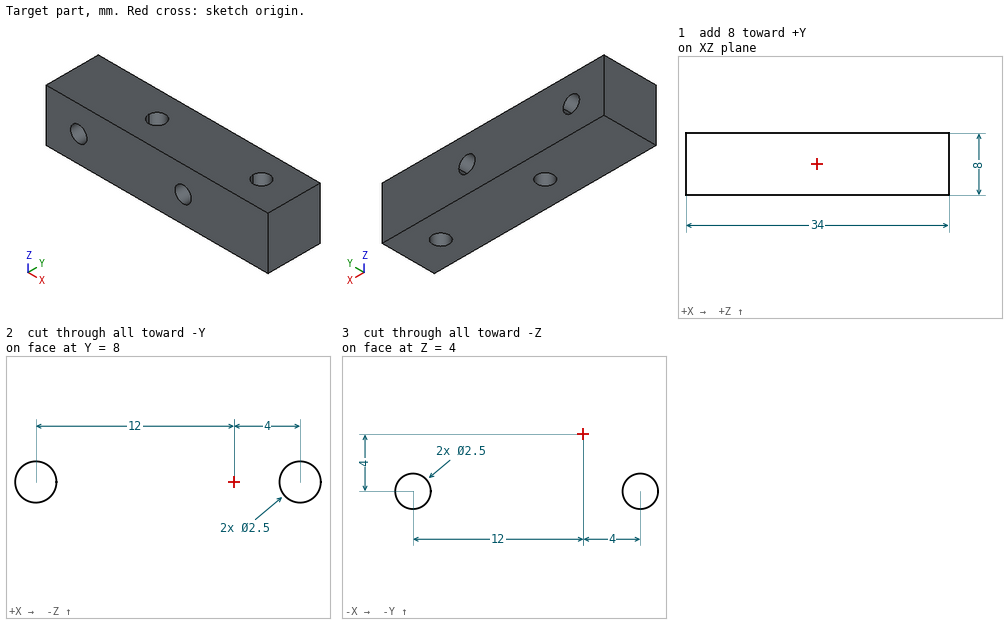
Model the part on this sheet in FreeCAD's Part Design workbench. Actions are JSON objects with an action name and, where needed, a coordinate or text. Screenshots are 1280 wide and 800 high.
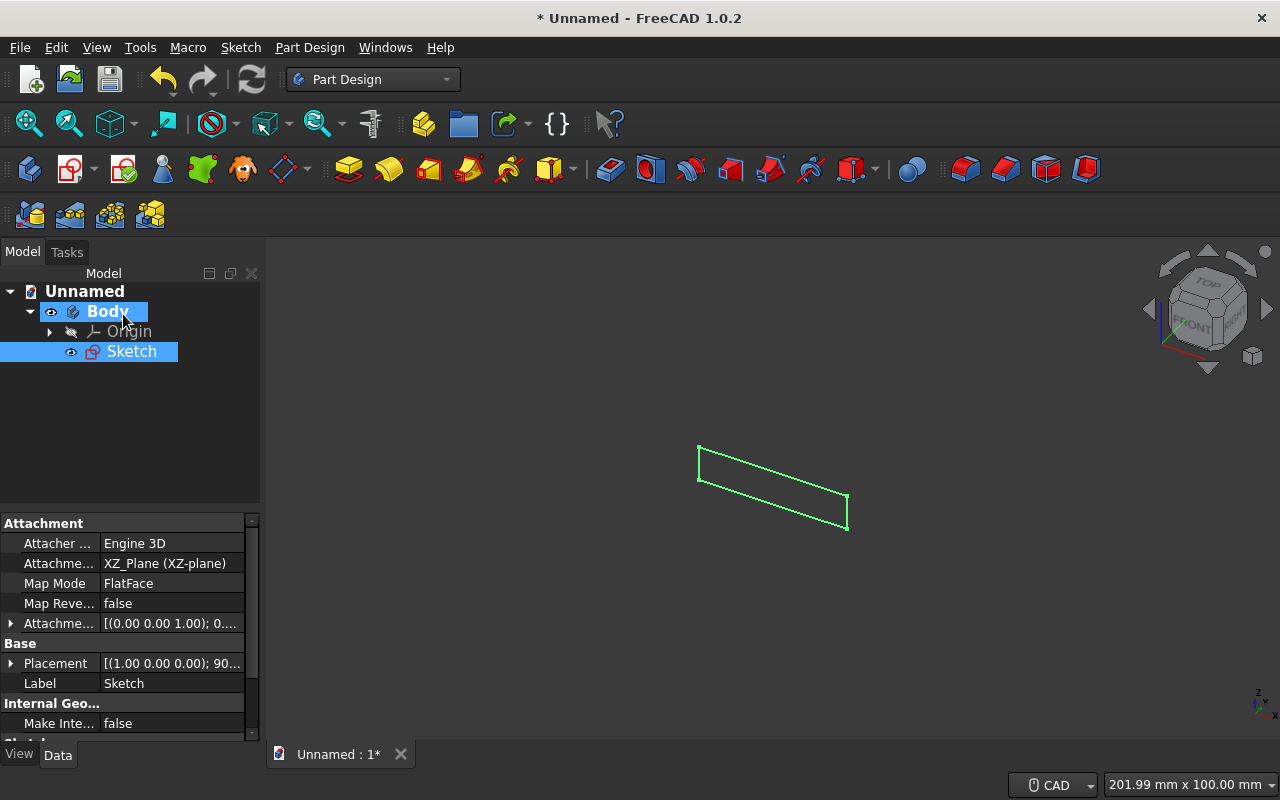
{"action": "left_click", "coordinate": [350, 170]}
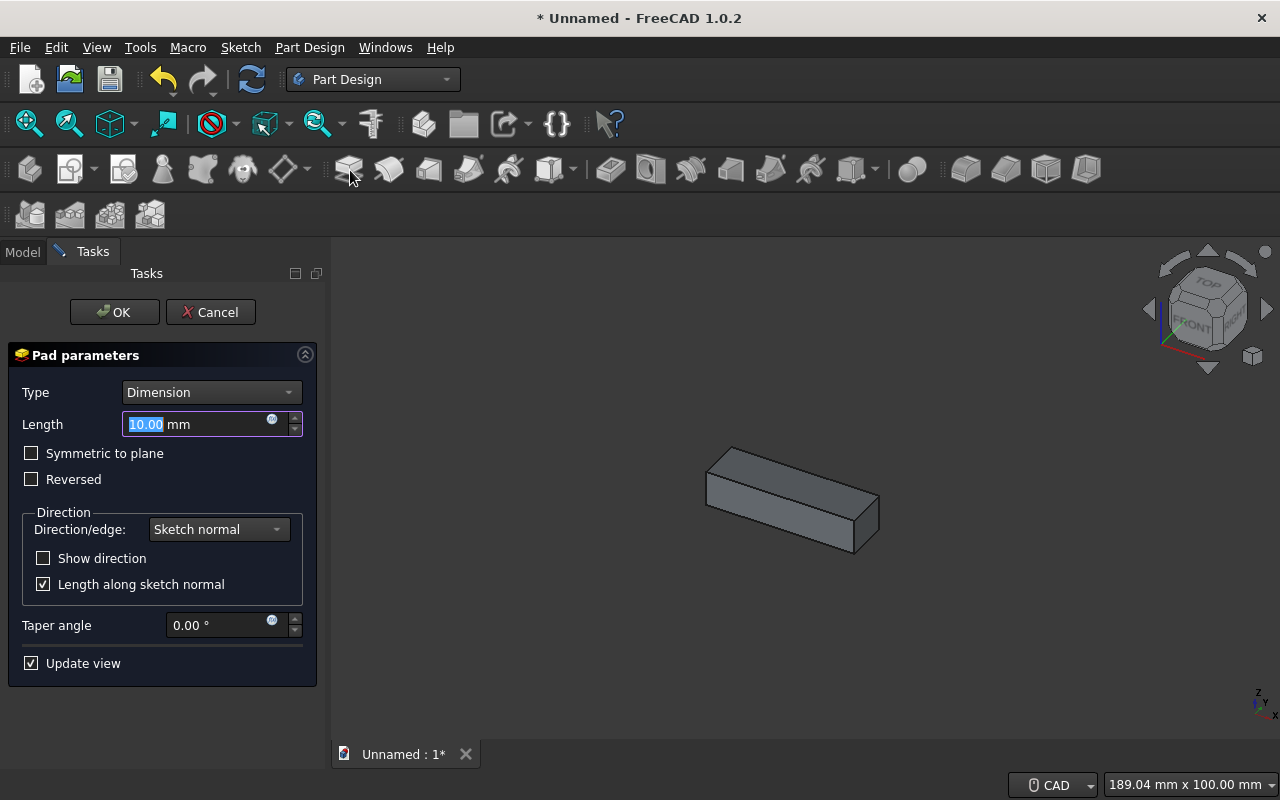
{"action": "type", "text": "8"}
{"action": "key", "text": "Tab"}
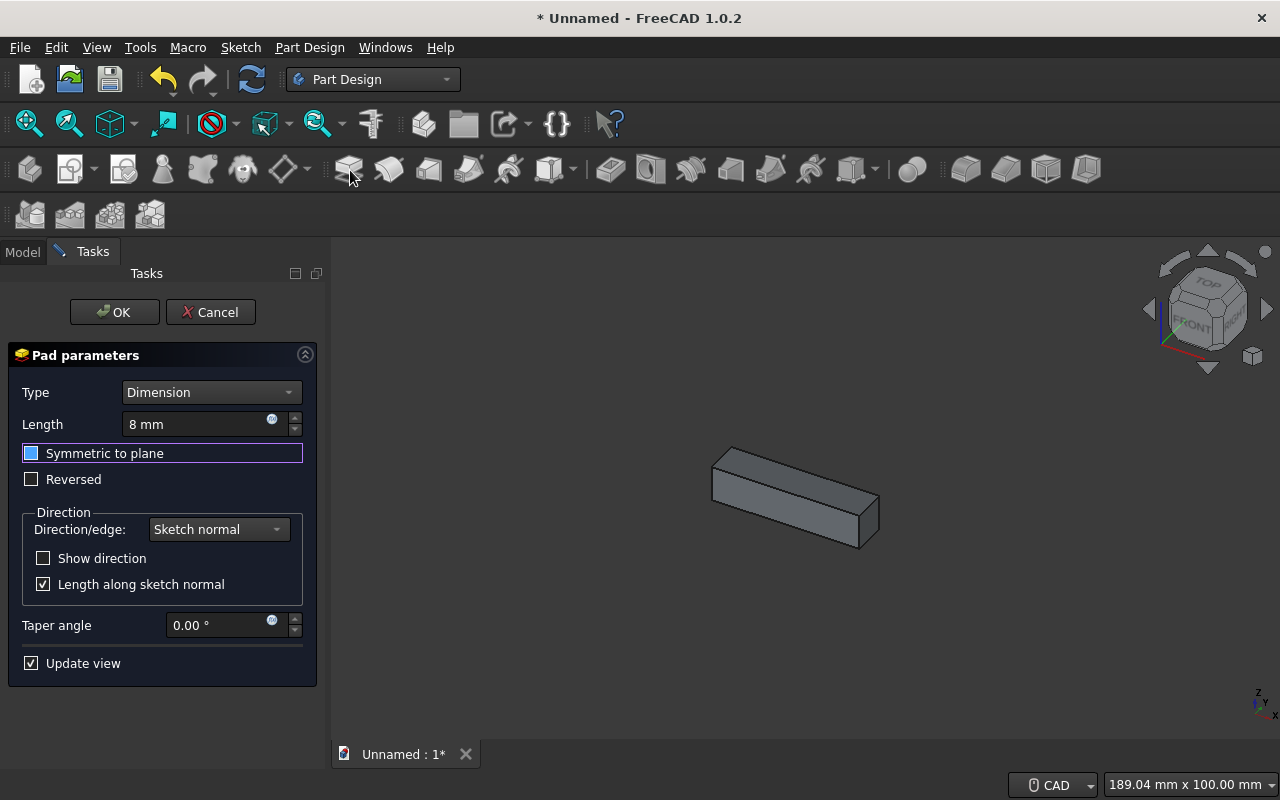
{"action": "left_click", "coordinate": [30, 479]}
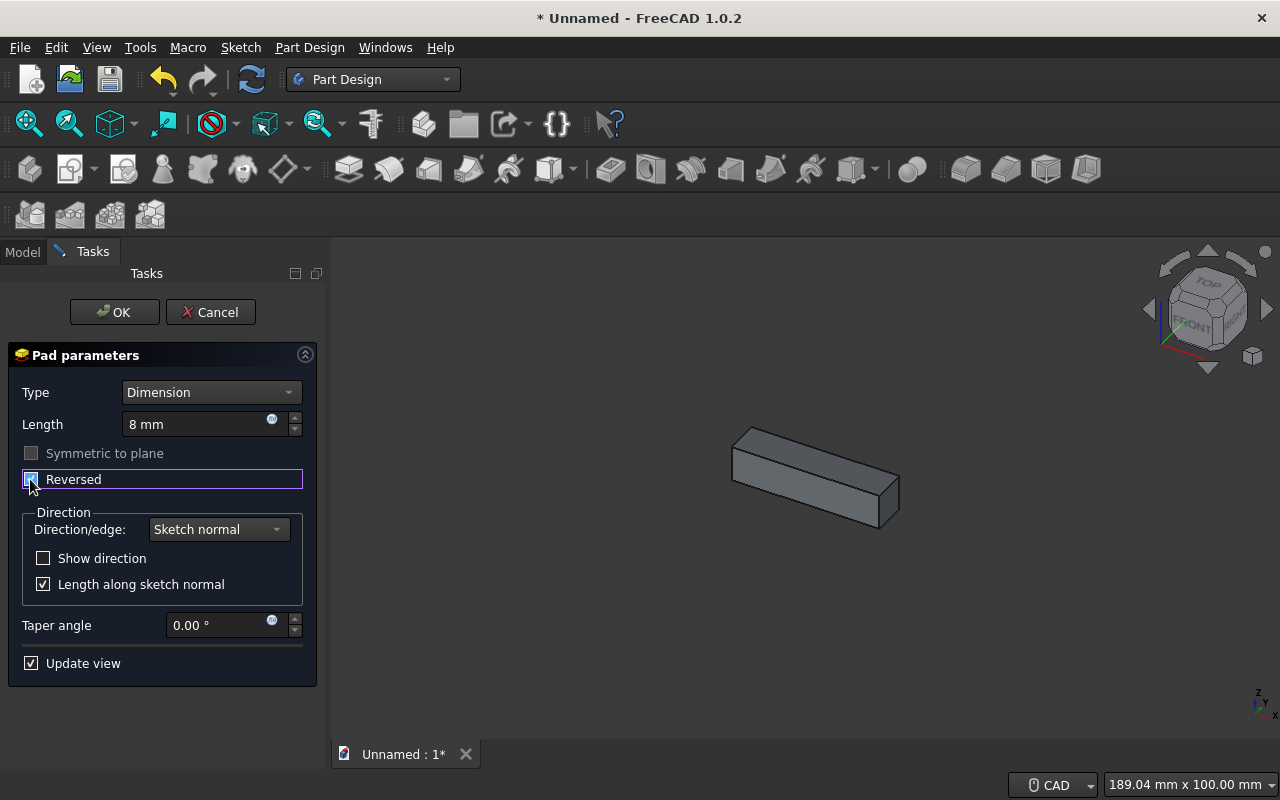
{"action": "left_click", "coordinate": [115, 312]}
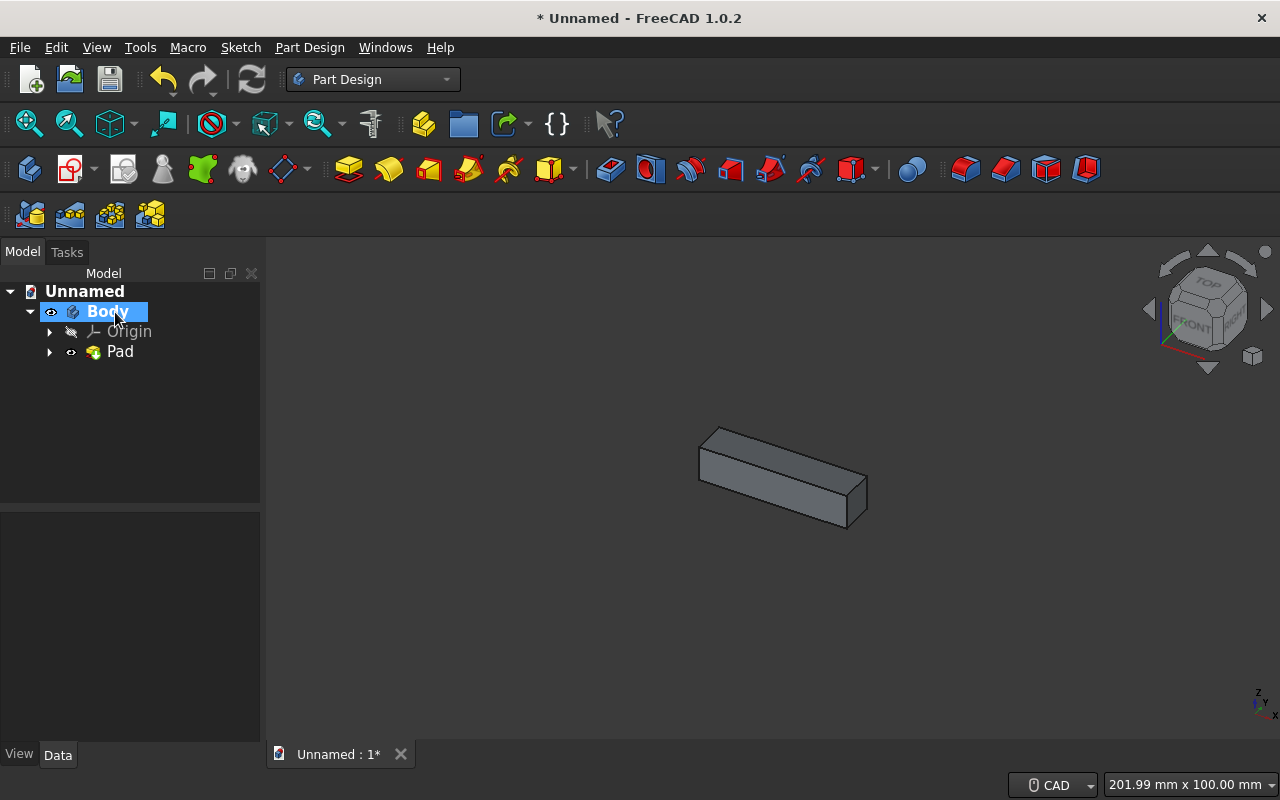
{"action": "left_click", "coordinate": [30, 124]}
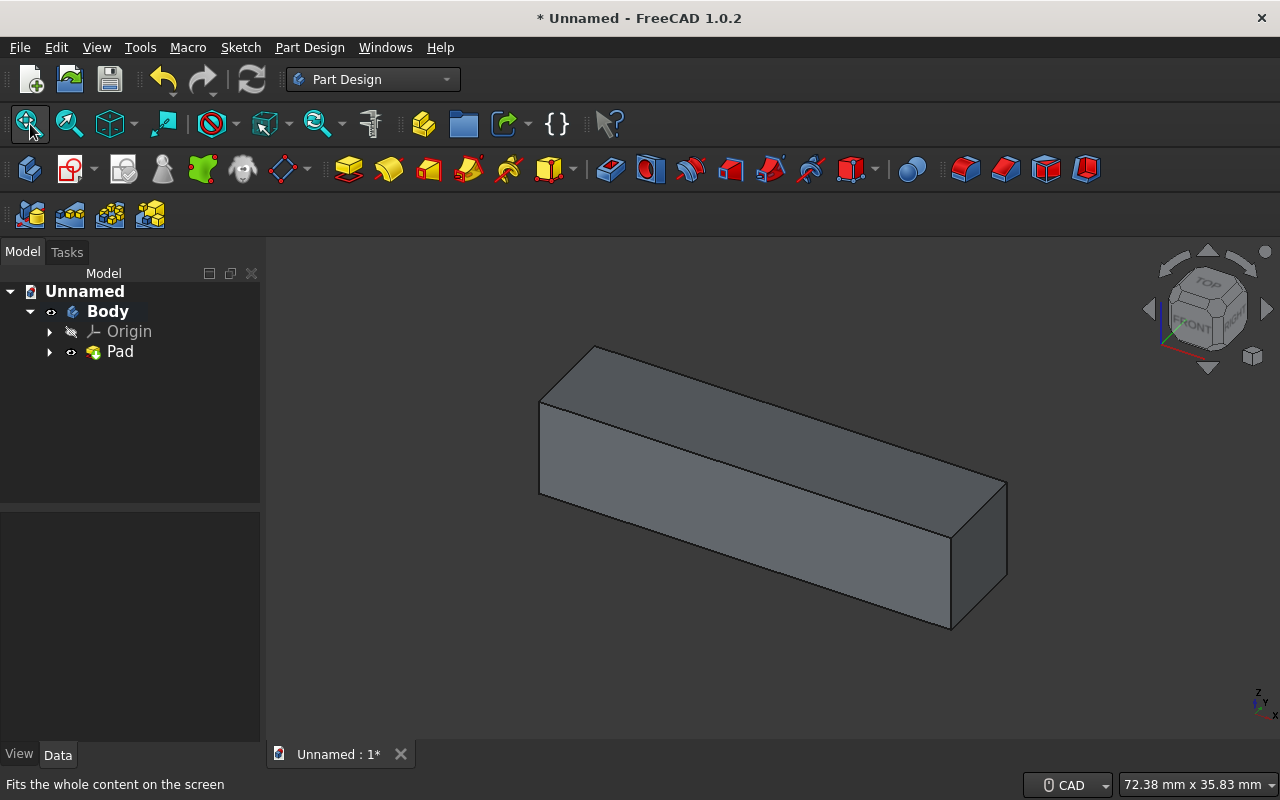
{"action": "key", "text": "4"}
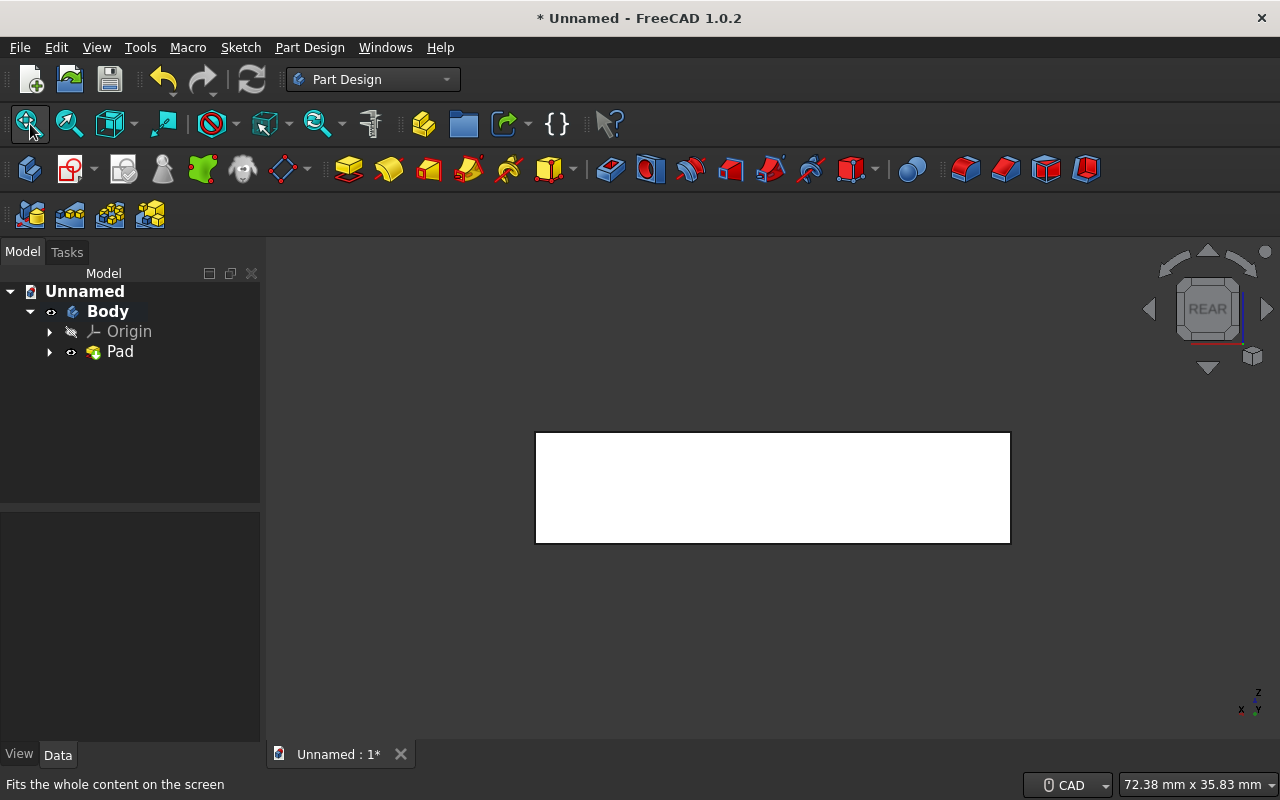
{"action": "left_click", "coordinate": [637, 487]}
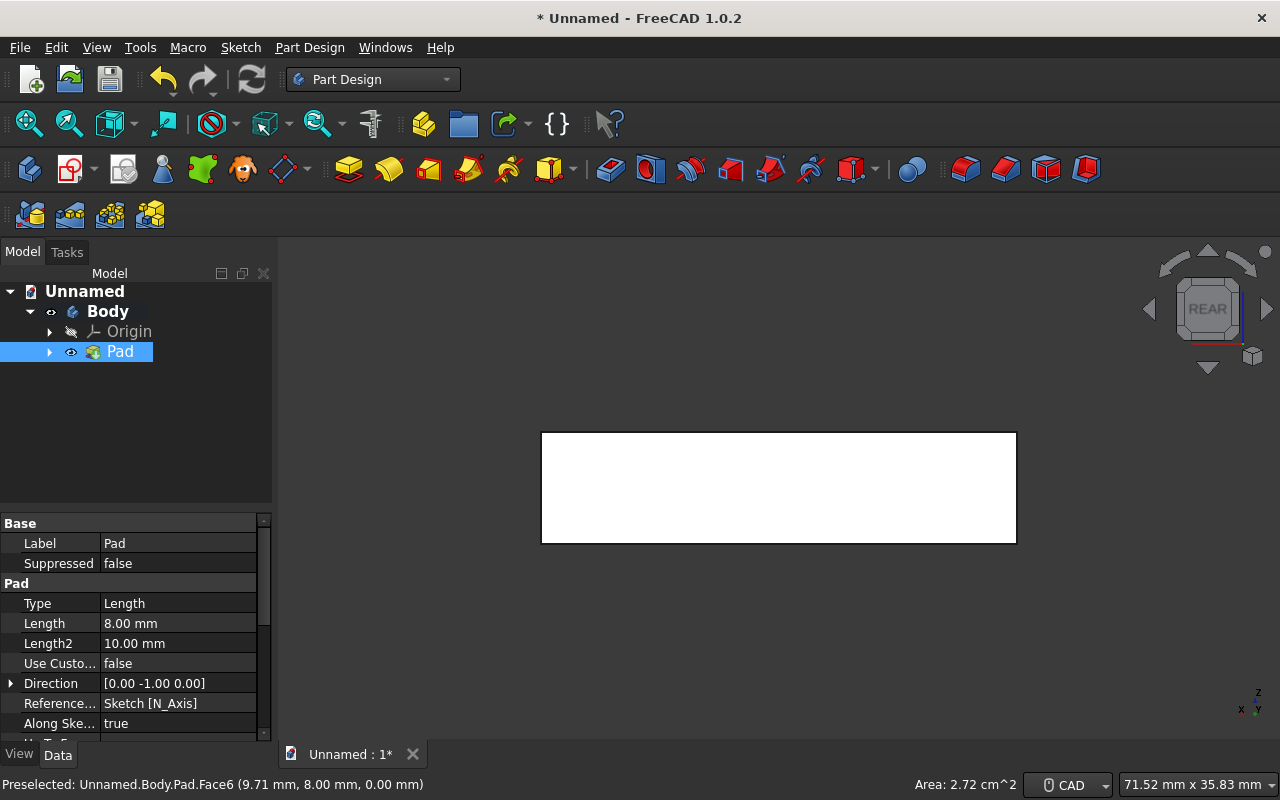
{"action": "left_click", "coordinate": [70, 170]}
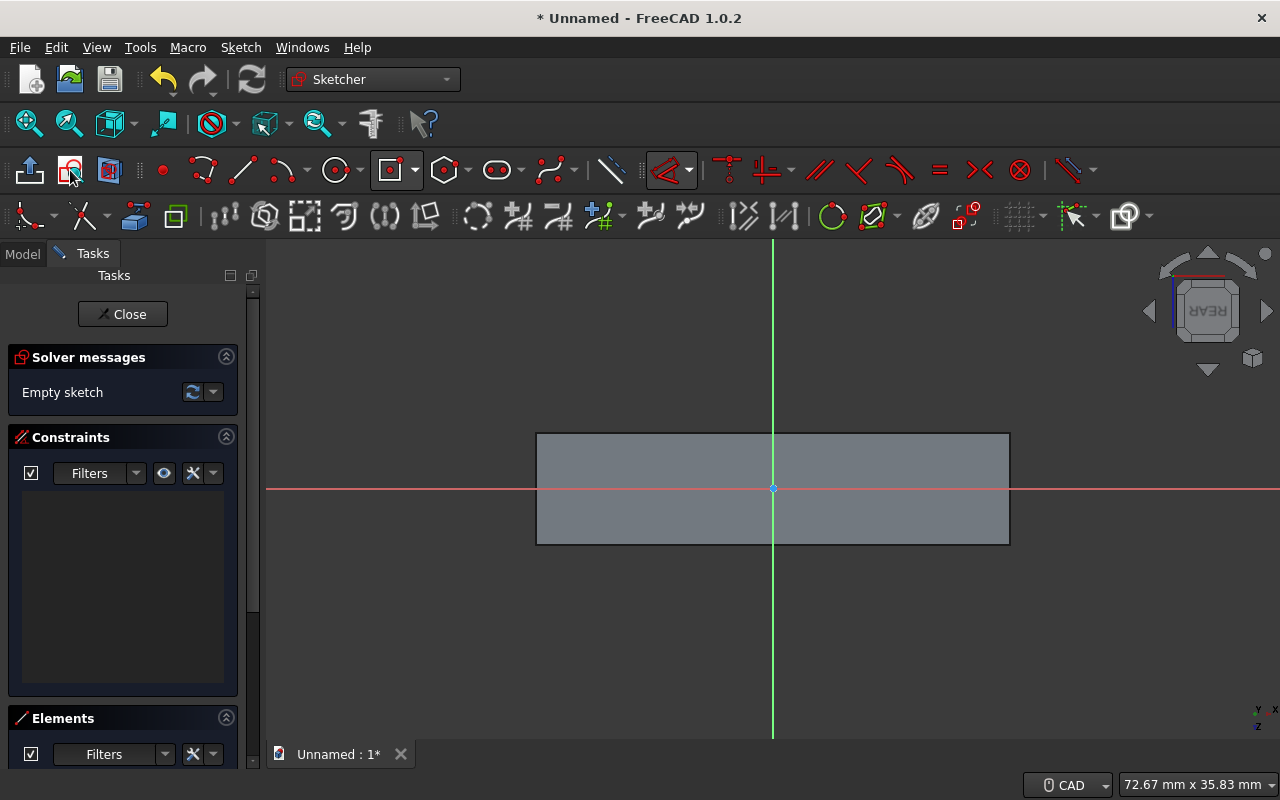
{"action": "scroll", "coordinate": [728, 489], "scroll_direction": "up", "scroll_amount": 4}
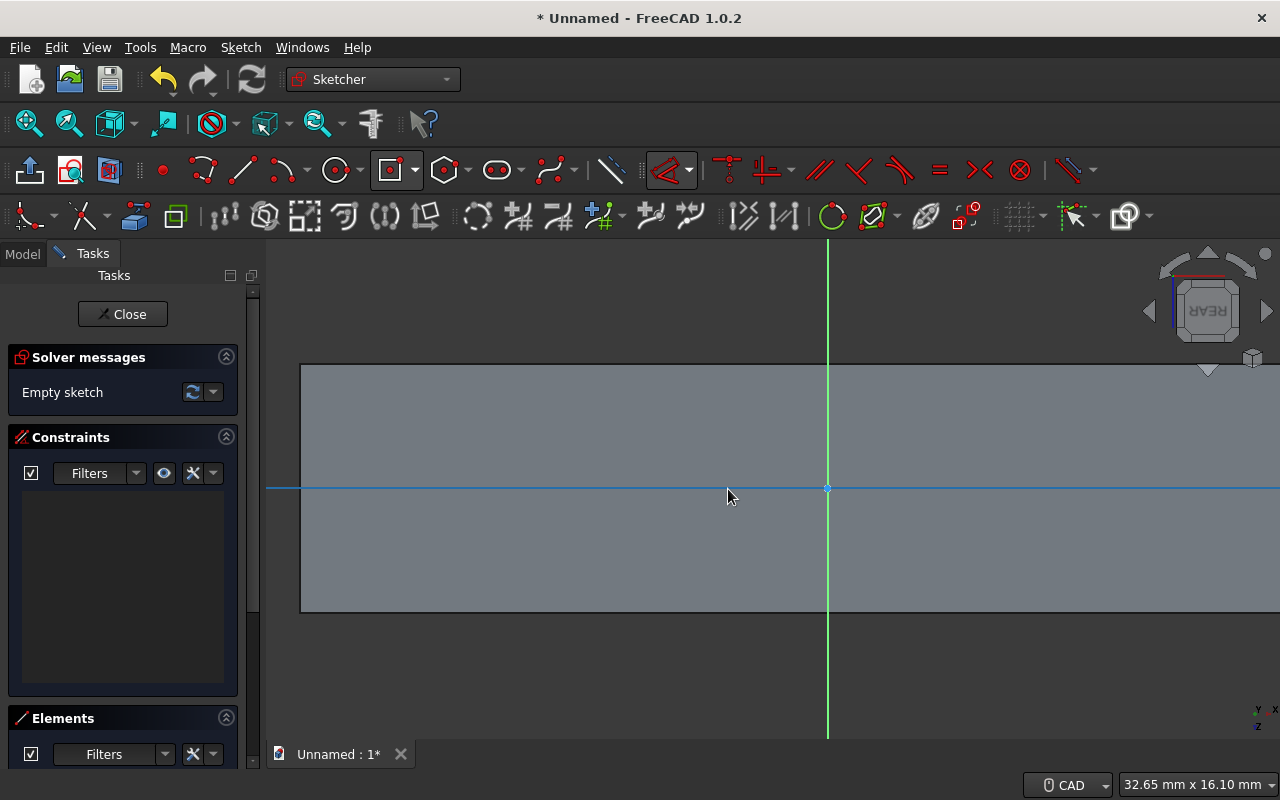
{"action": "left_click", "coordinate": [336, 170]}